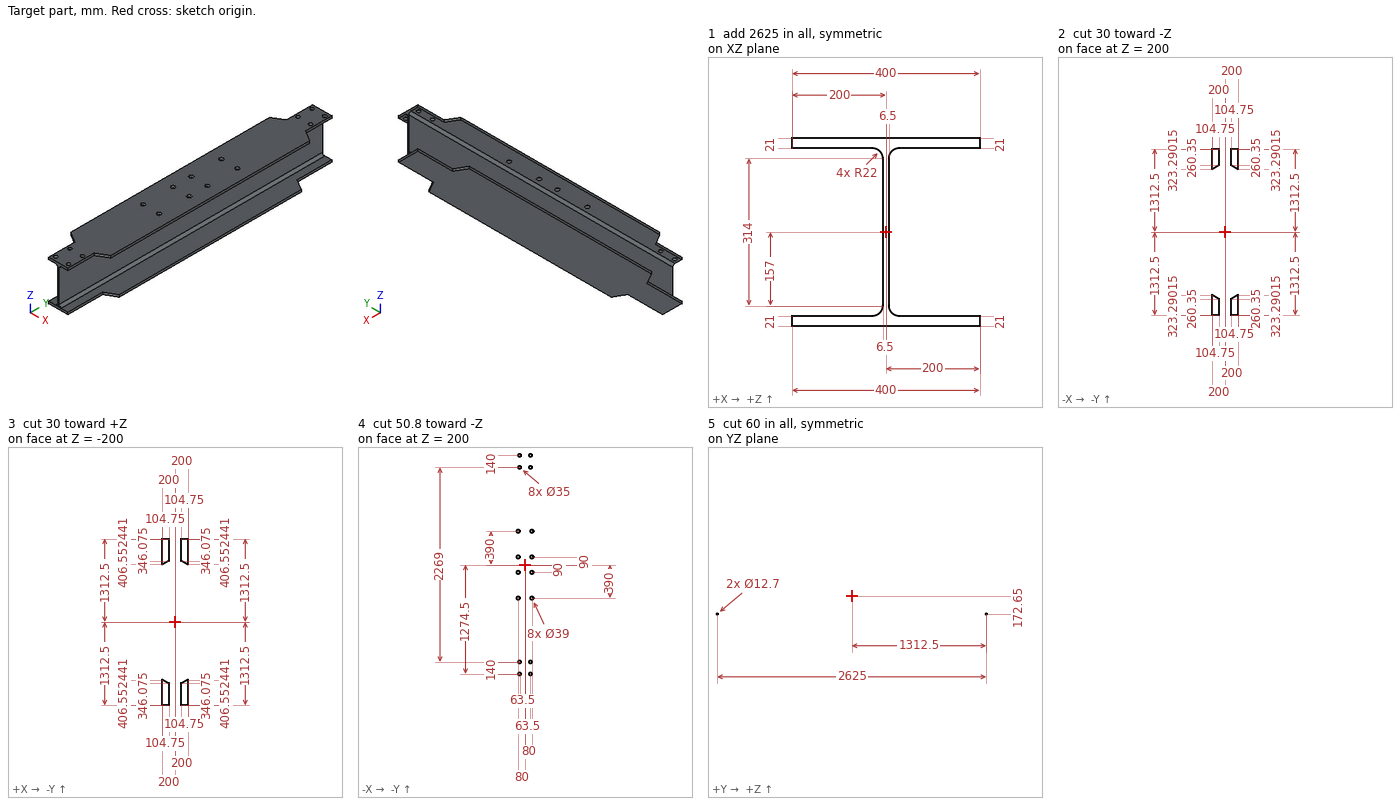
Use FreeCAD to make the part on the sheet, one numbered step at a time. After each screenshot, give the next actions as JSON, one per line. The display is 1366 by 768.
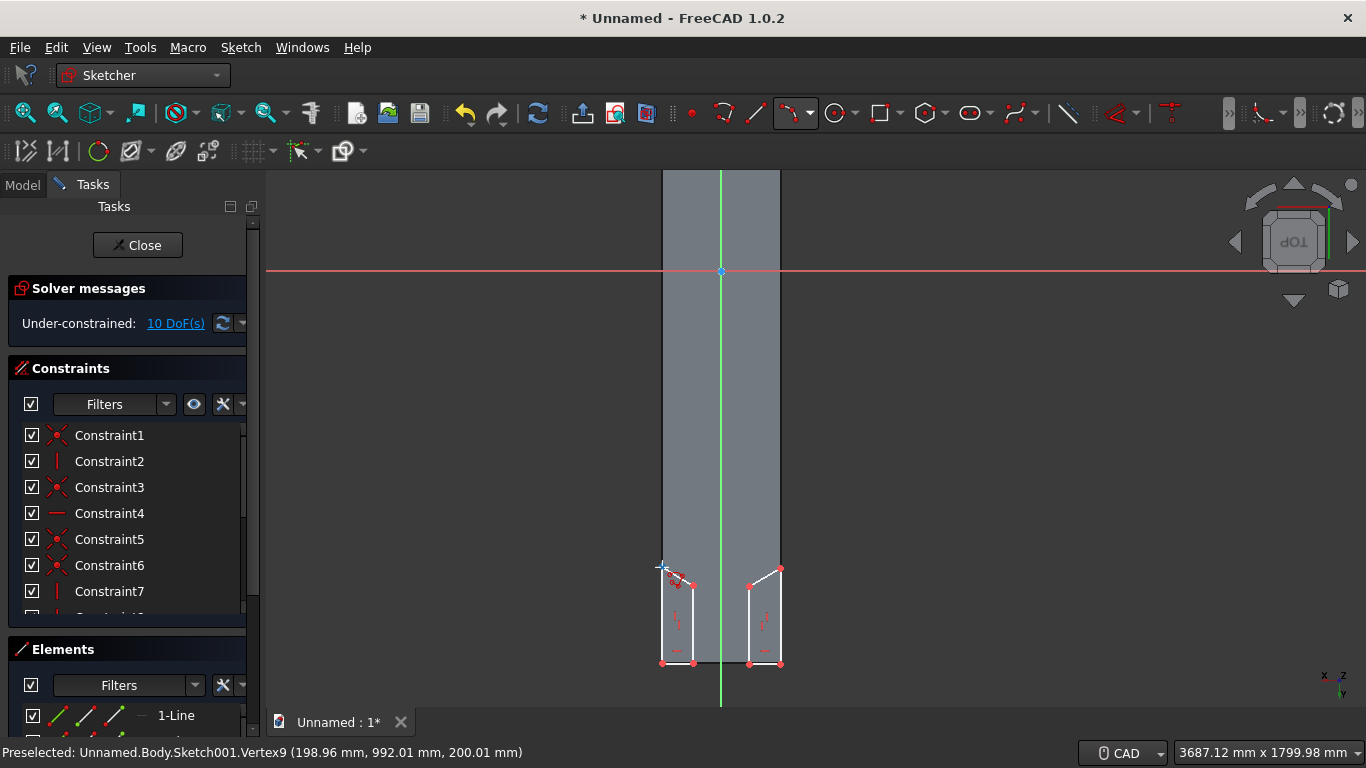
{"action": "scroll", "coordinate": [769, 575], "scroll_direction": "down", "scroll_amount": 4}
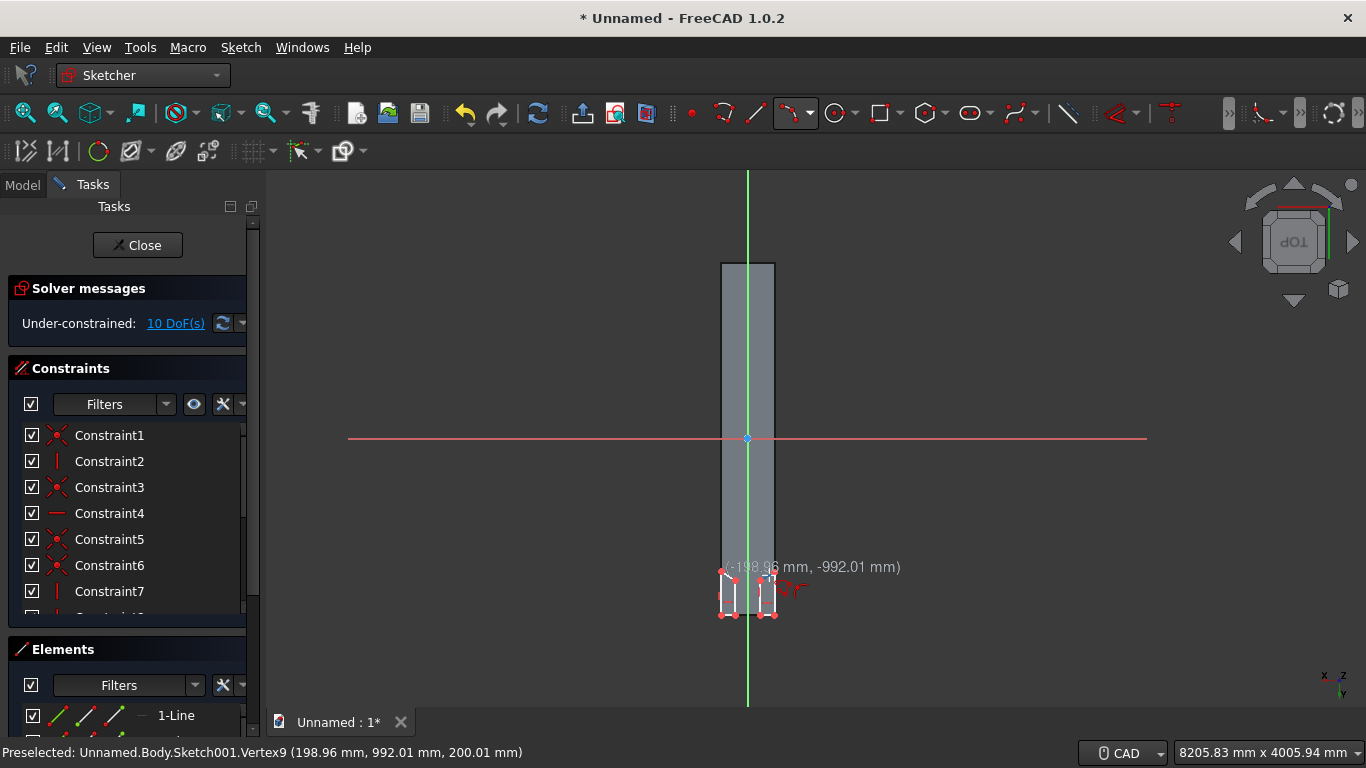
{"action": "left_click", "coordinate": [721, 306]}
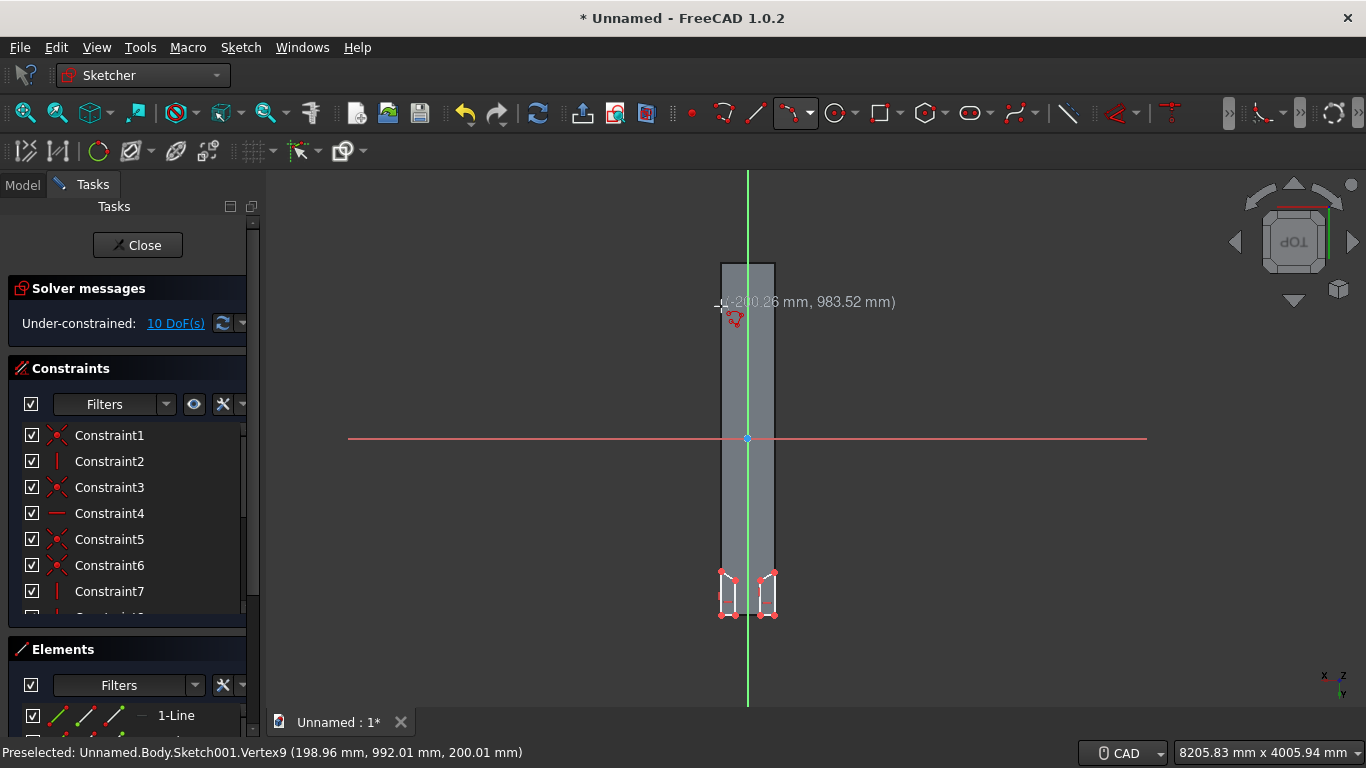
{"action": "scroll", "coordinate": [735, 298], "scroll_direction": "up", "scroll_amount": 2}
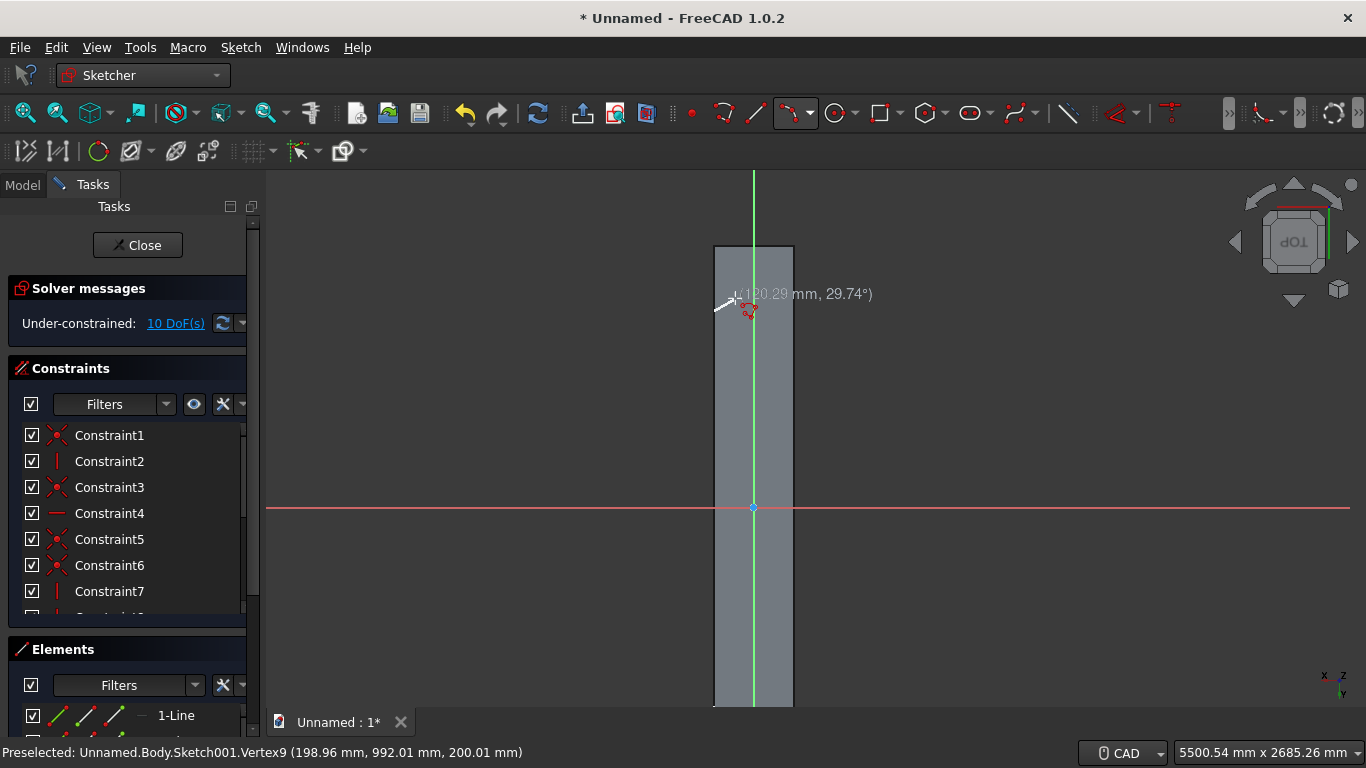
{"action": "left_click", "coordinate": [735, 298]}
{"action": "left_click", "coordinate": [735, 246]}
{"action": "left_click", "coordinate": [714, 246]}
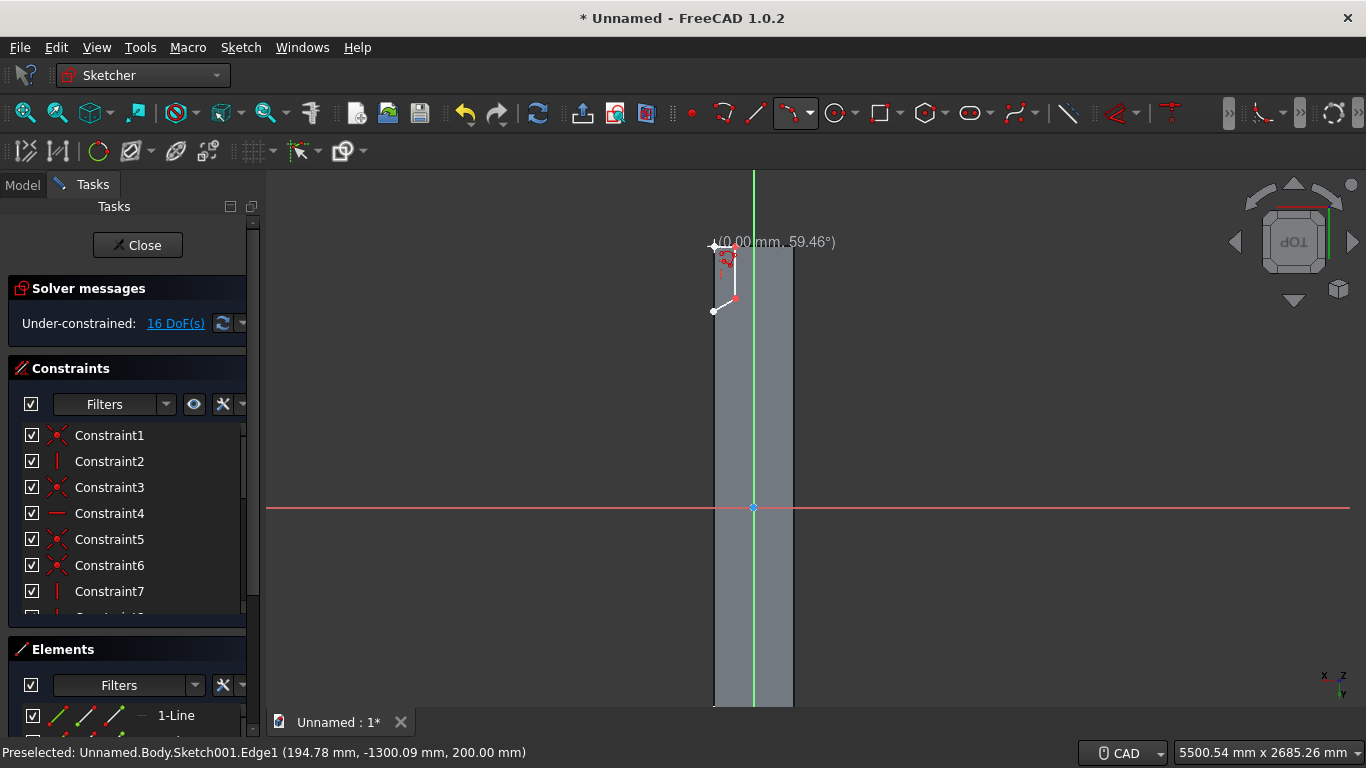
{"action": "scroll", "coordinate": [714, 310], "scroll_direction": "up", "scroll_amount": 2}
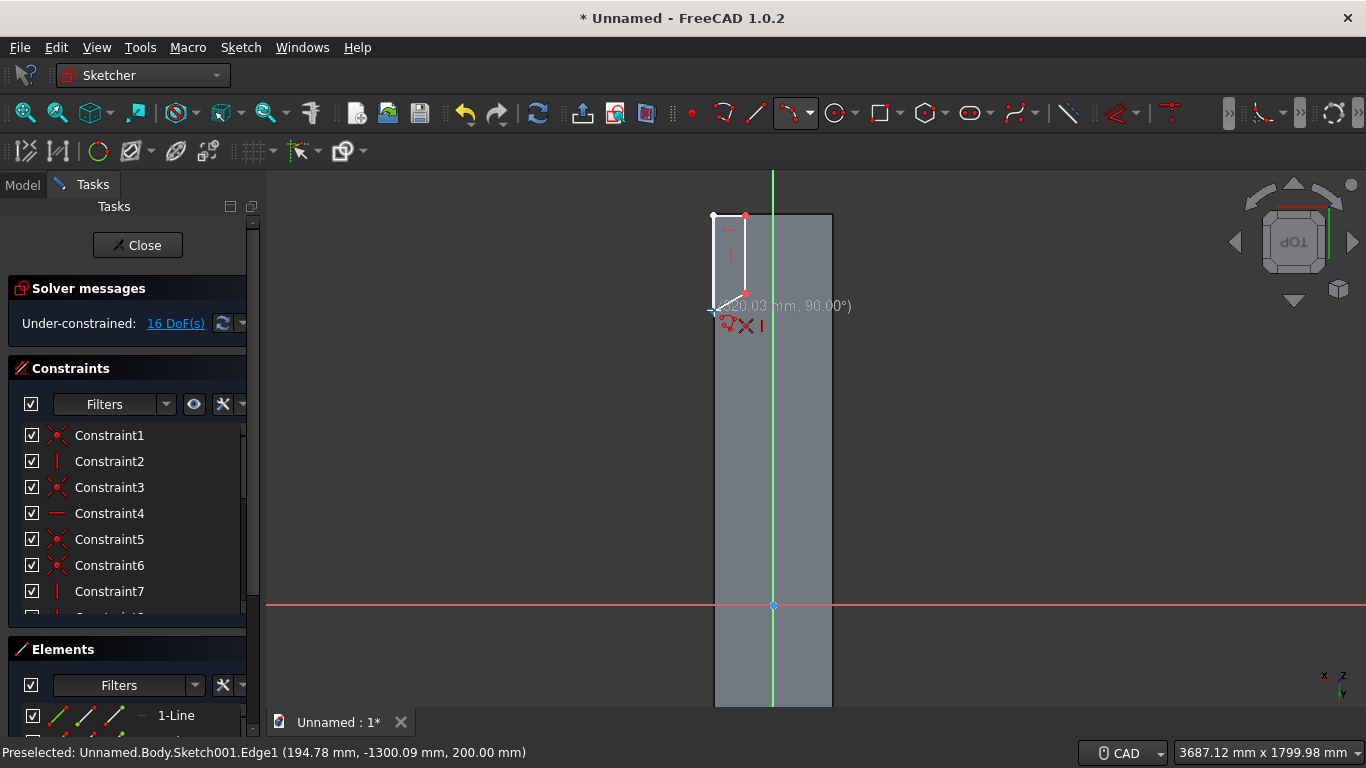
{"action": "left_click", "coordinate": [714, 312]}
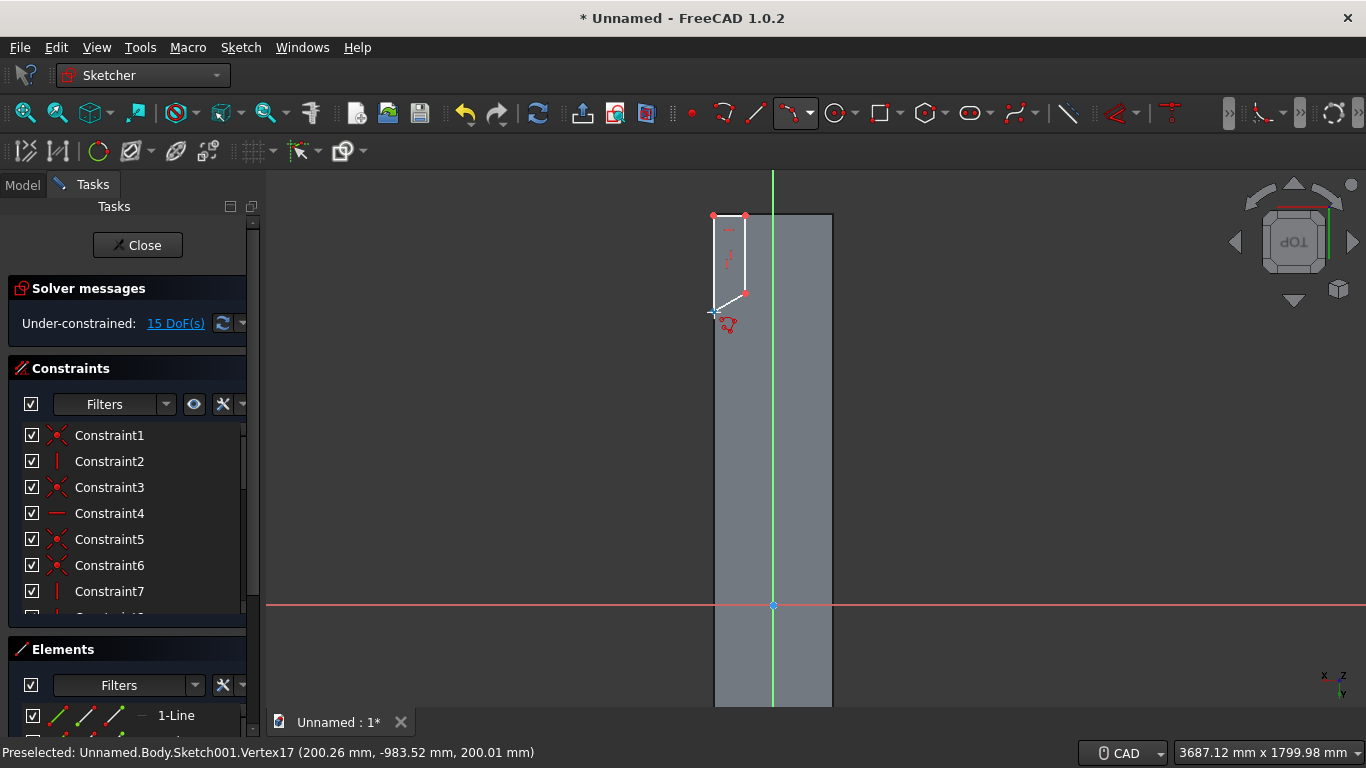
{"action": "left_click", "coordinate": [833, 310]}
{"action": "left_click", "coordinate": [833, 214]}
{"action": "left_click", "coordinate": [802, 214]}
{"action": "left_click", "coordinate": [802, 291]}
{"action": "left_click", "coordinate": [833, 311]}
{"action": "key", "text": "Escape"}
{"action": "key", "text": "Escape"}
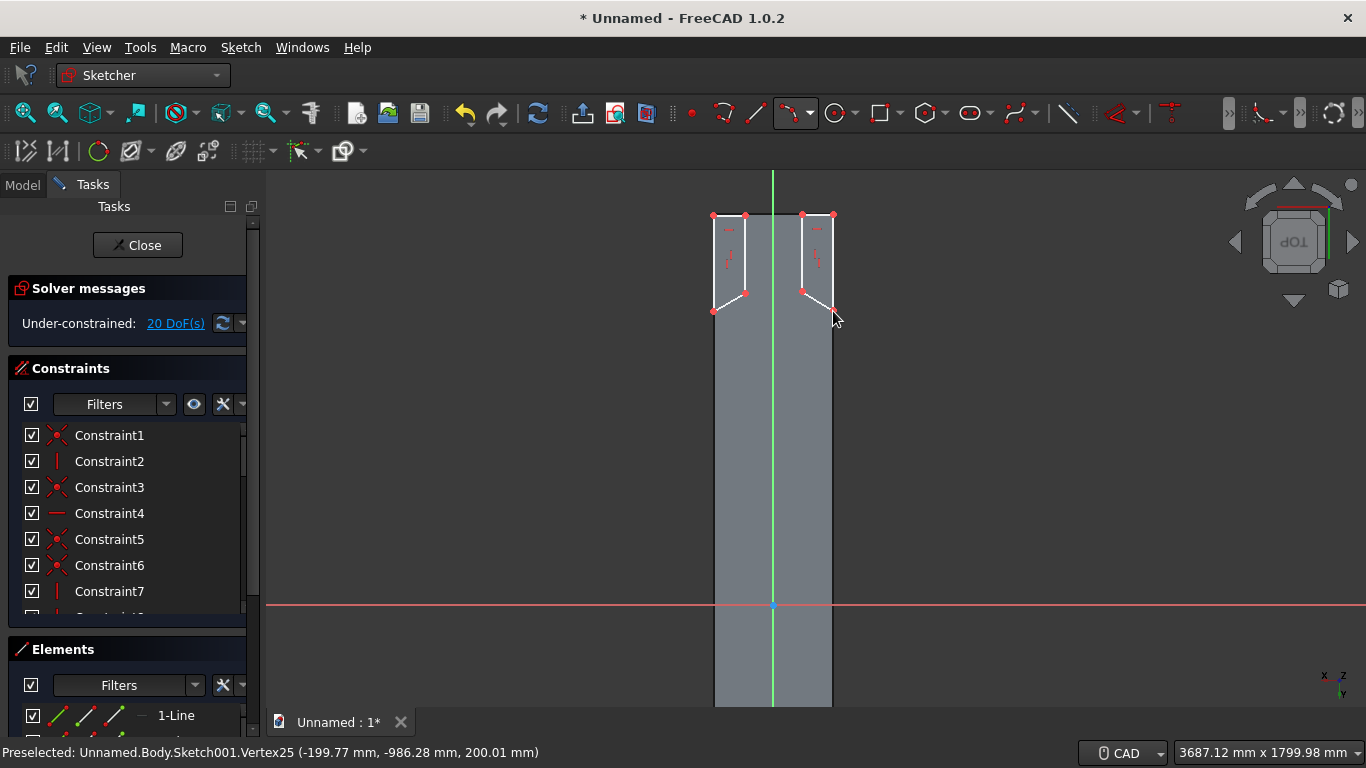
{"action": "left_click", "coordinate": [1116, 114]}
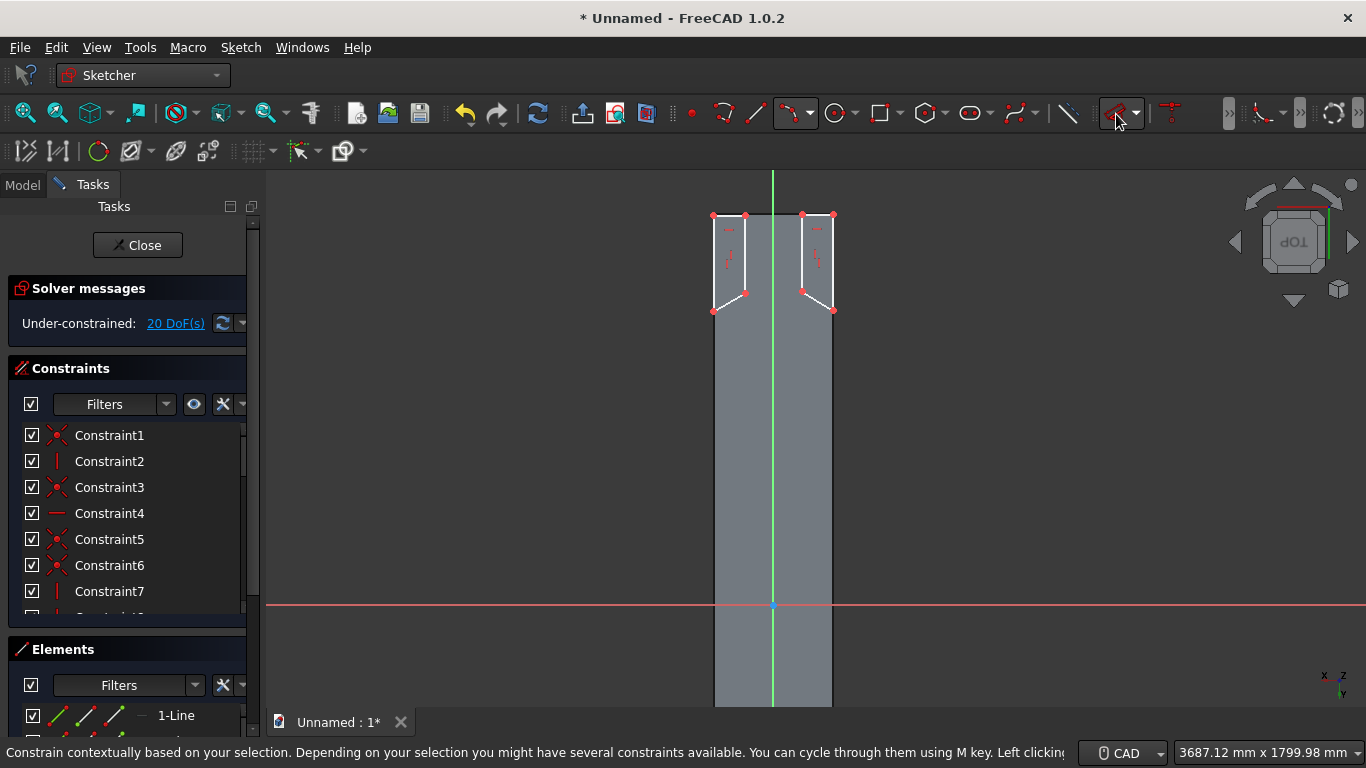
{"action": "scroll", "coordinate": [726, 302], "scroll_direction": "down", "scroll_amount": 4}